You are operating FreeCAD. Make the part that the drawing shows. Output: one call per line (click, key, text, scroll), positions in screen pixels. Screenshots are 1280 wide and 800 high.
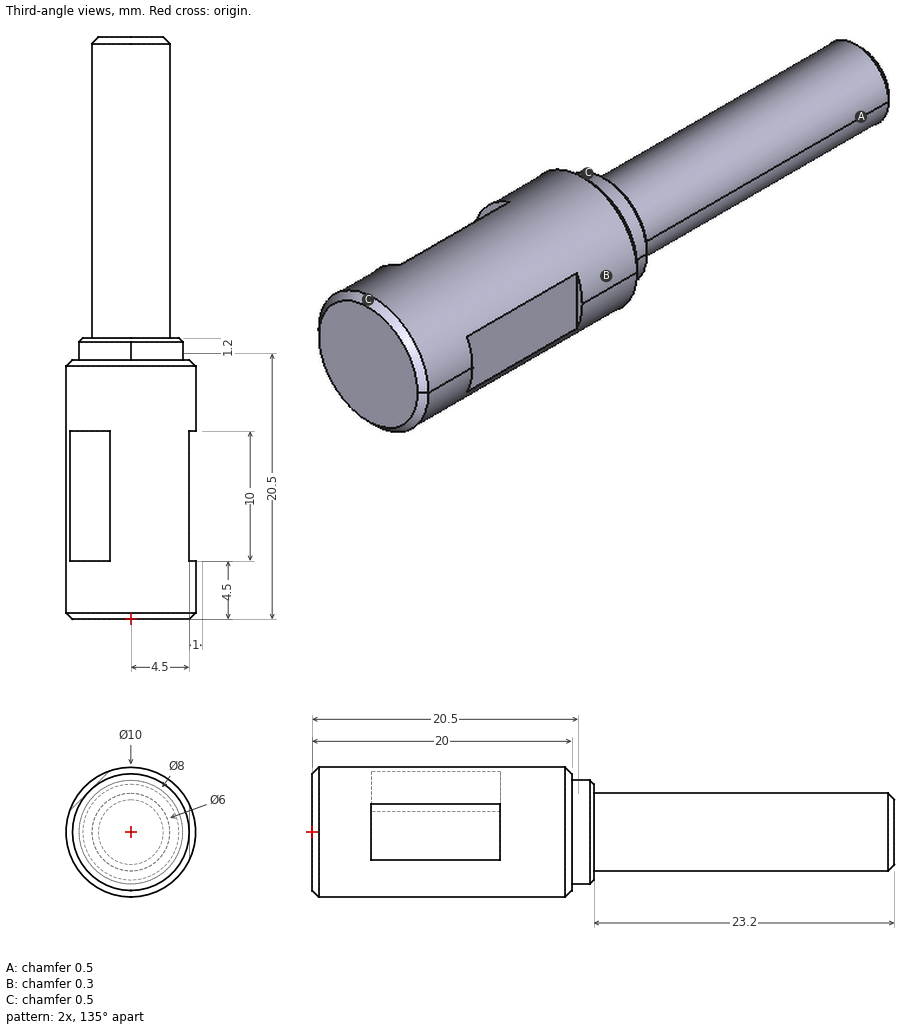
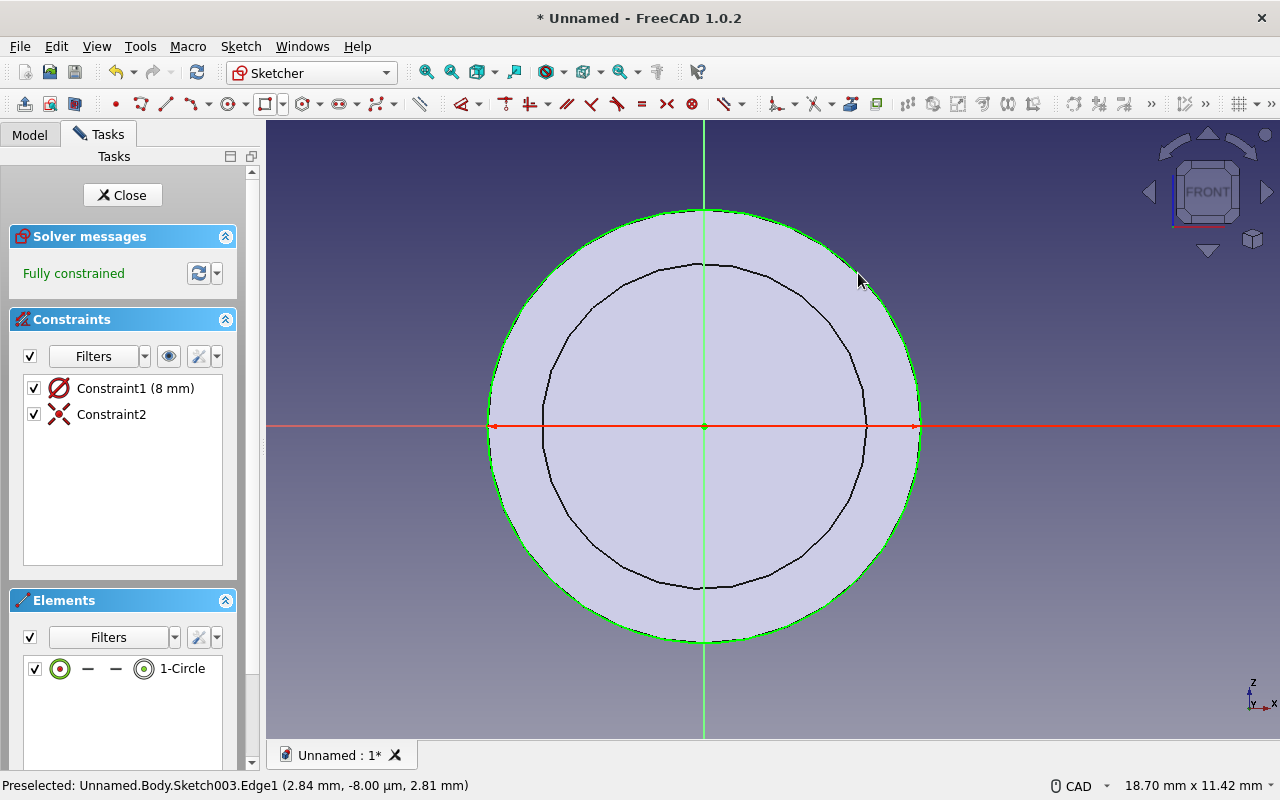
click(123, 195)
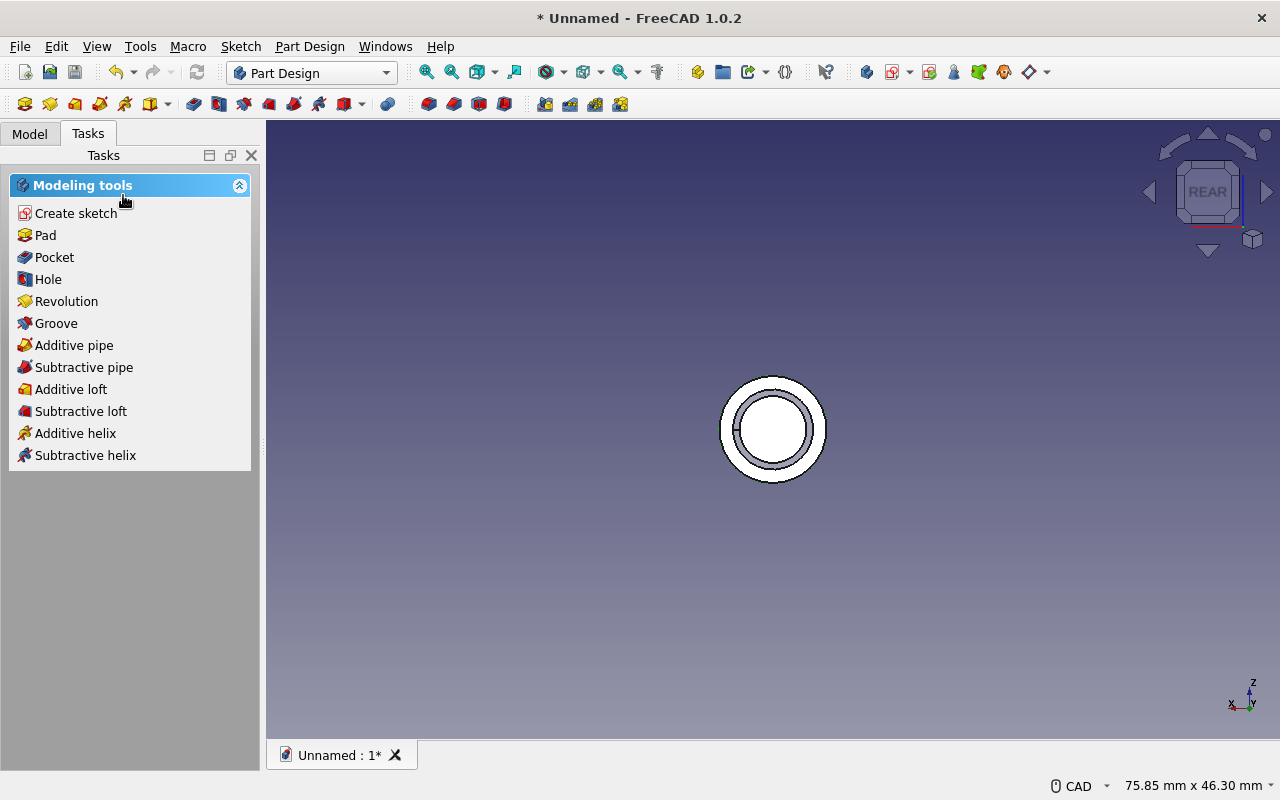
click(25, 104)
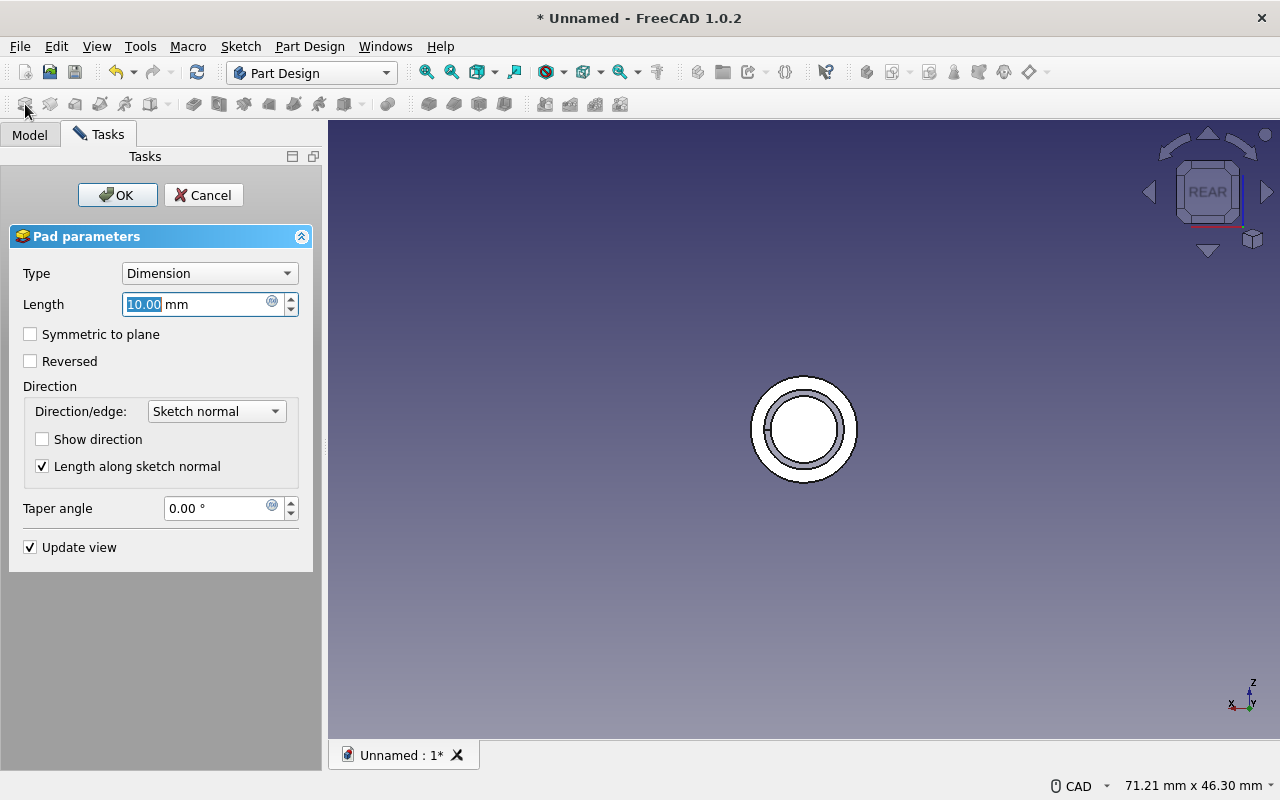
text(20.5)
key(Tab)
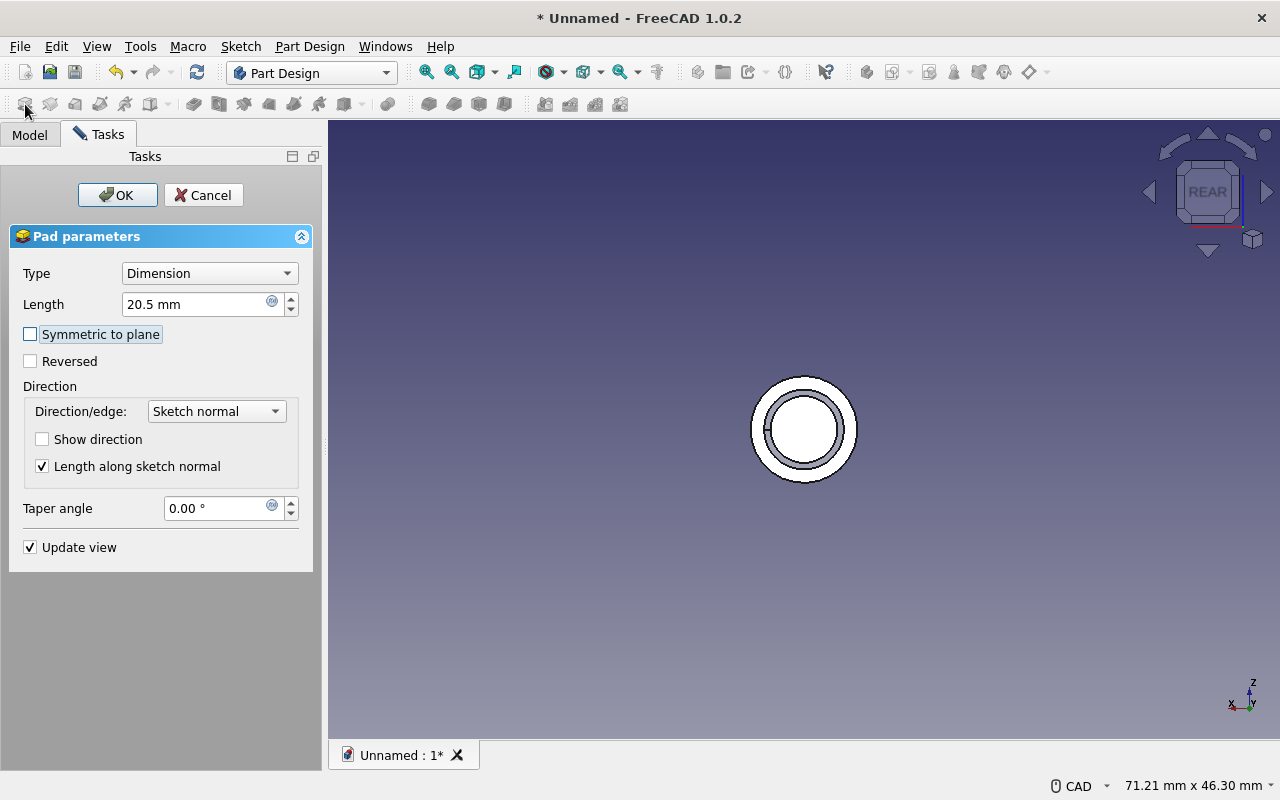
click(31, 361)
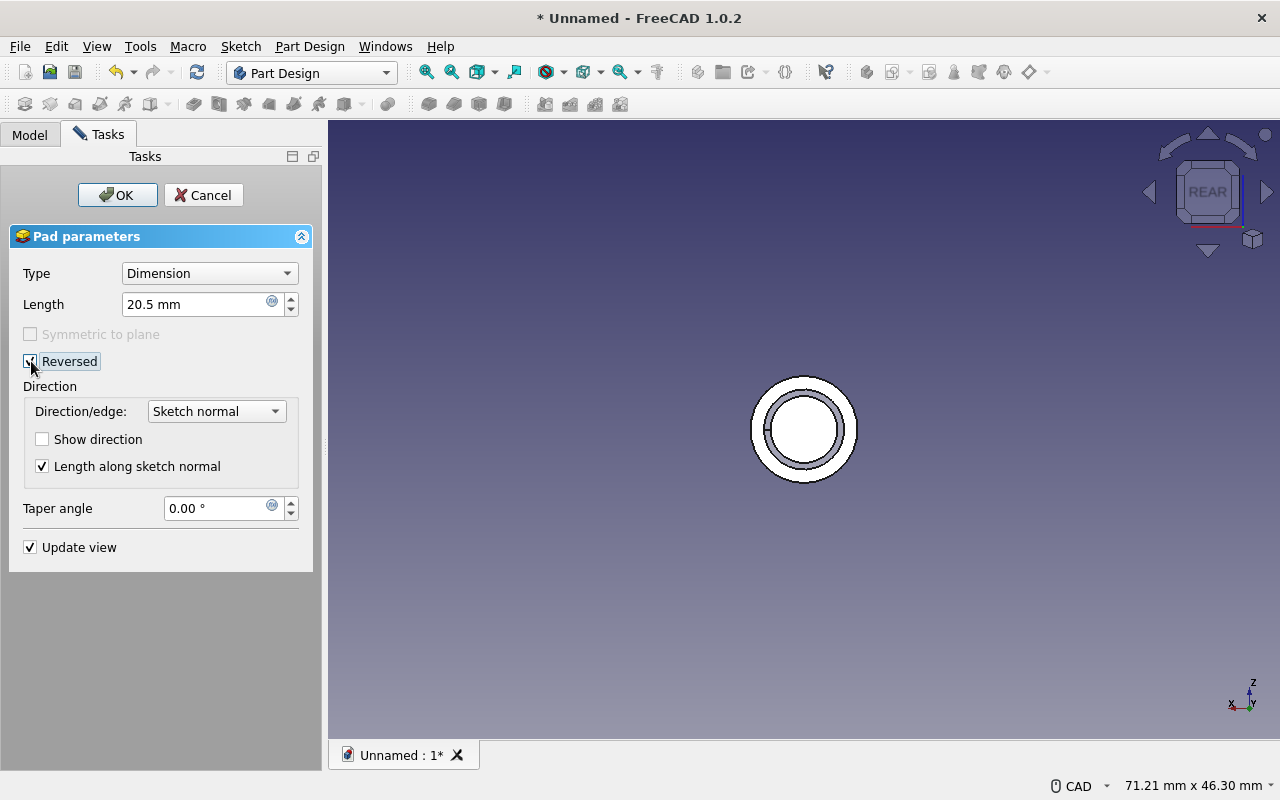
click(118, 195)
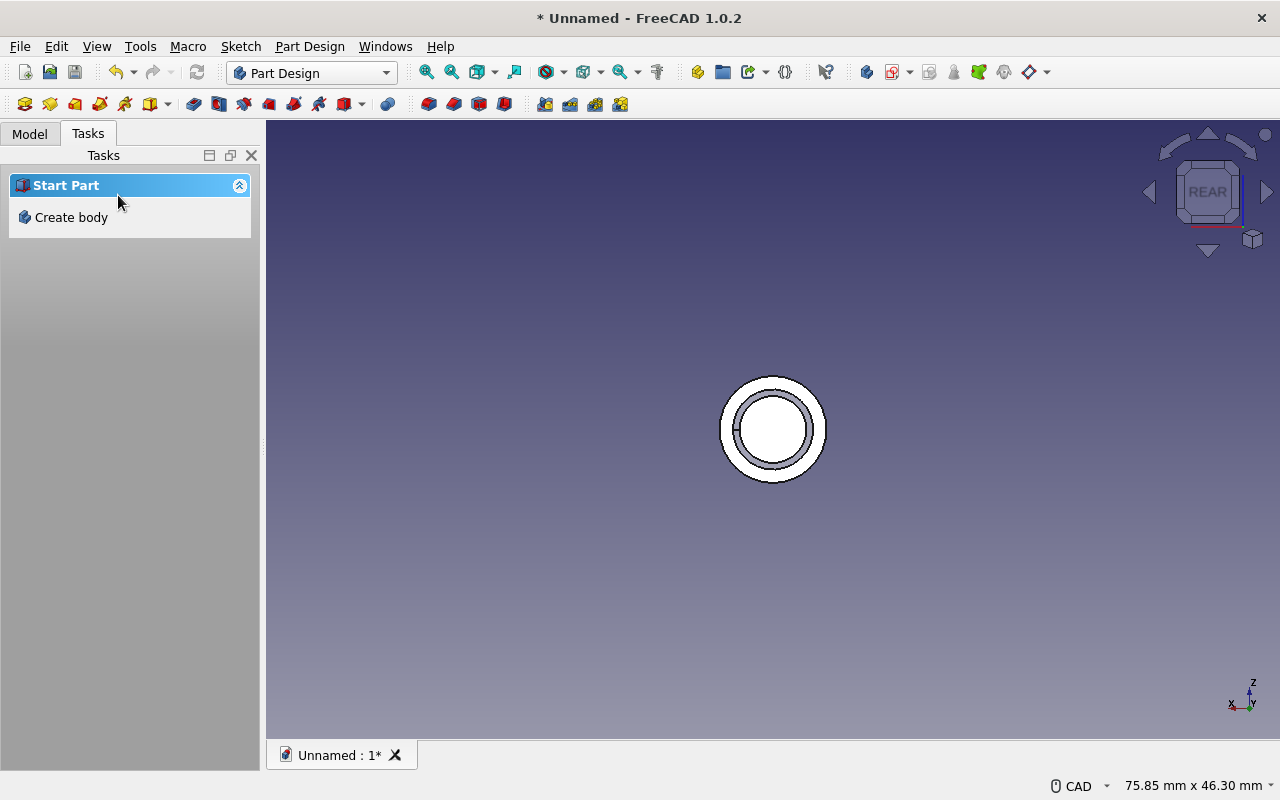
click(427, 72)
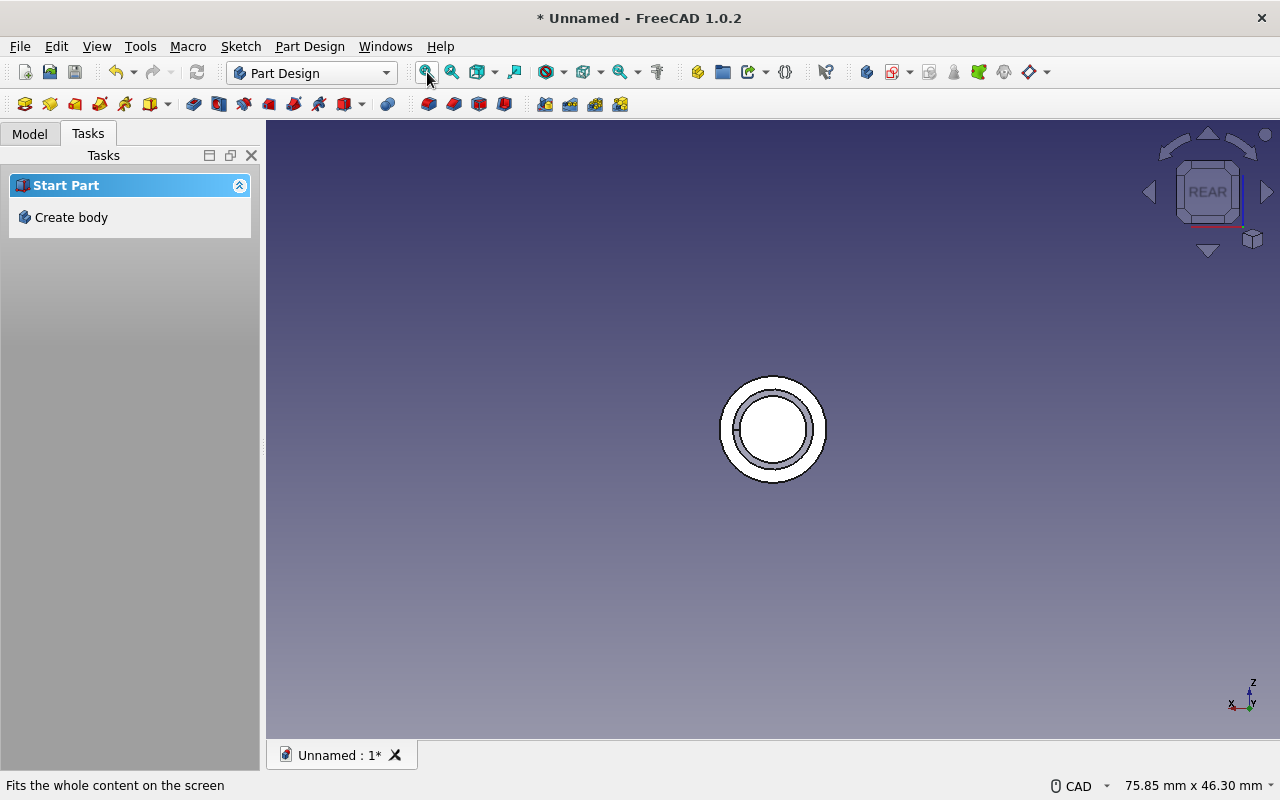
click(826, 428)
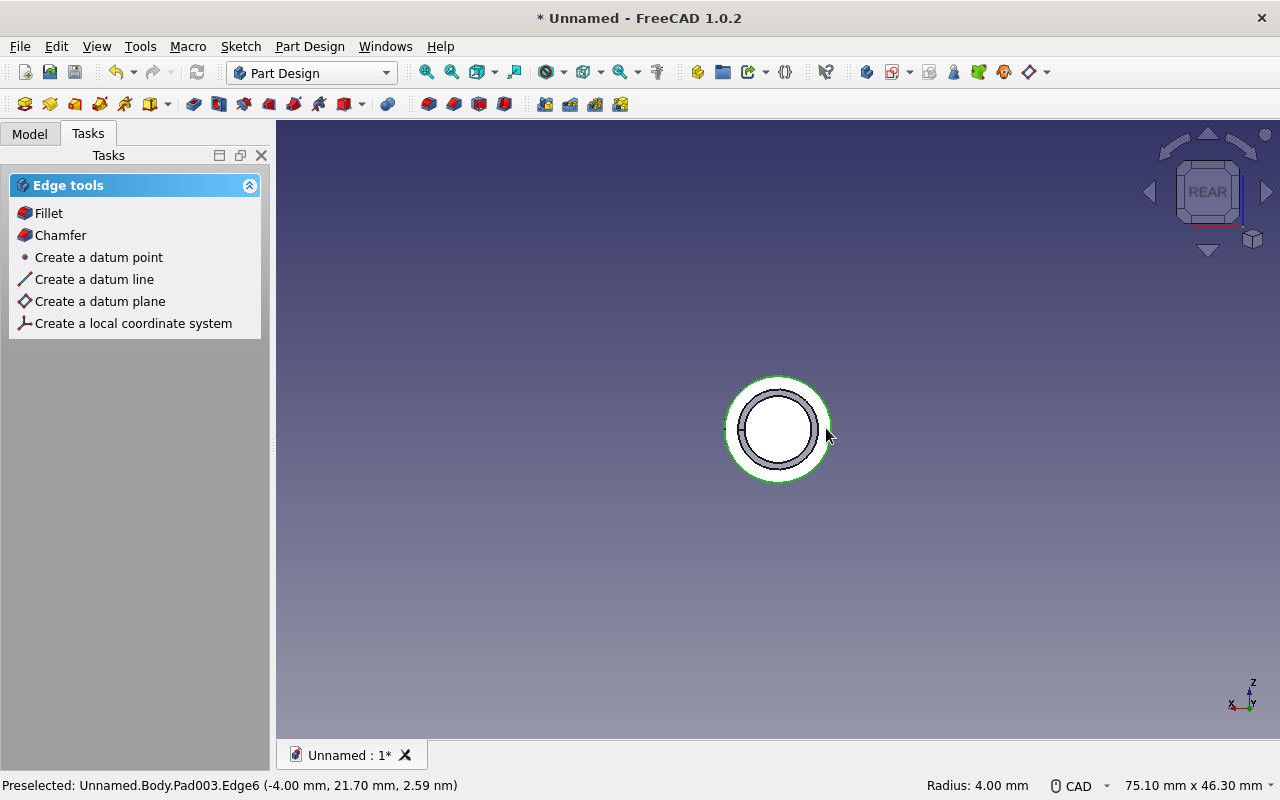
click(454, 104)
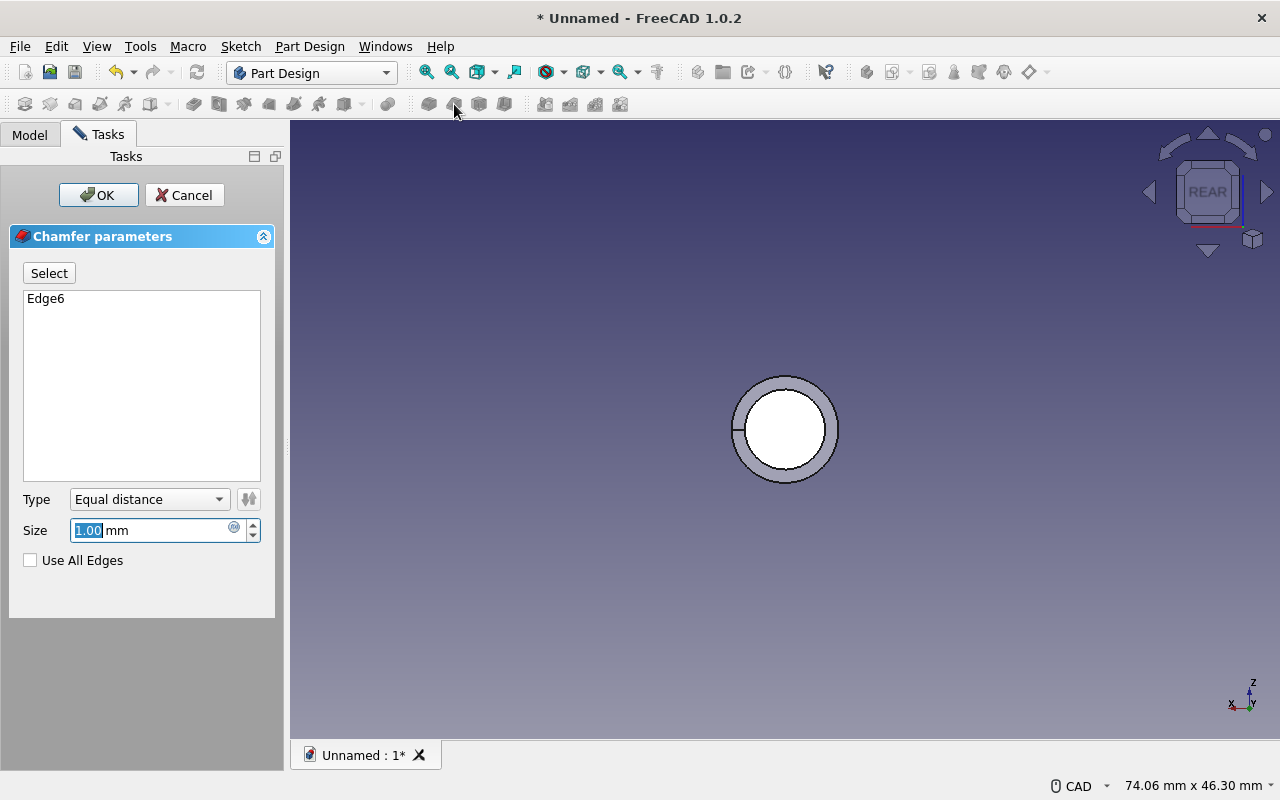
text(0.3)
key(Tab)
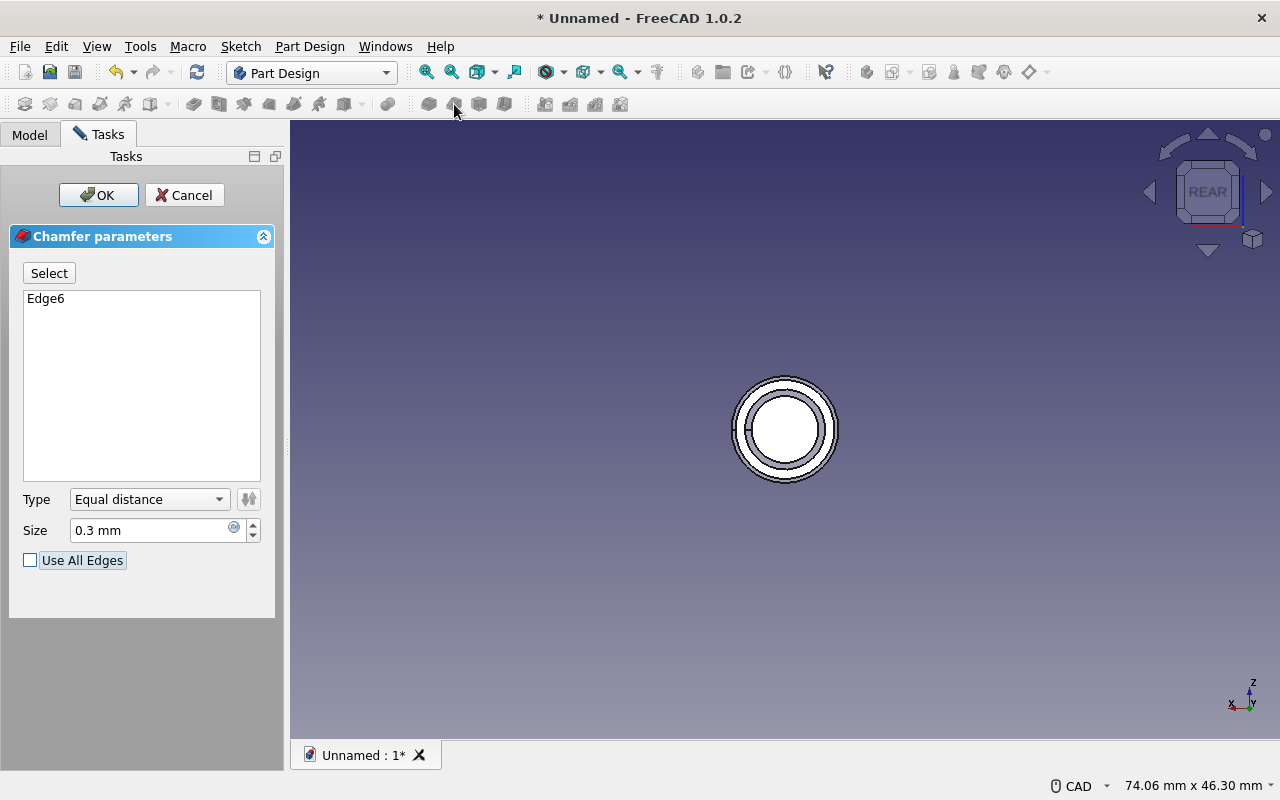
click(99, 195)